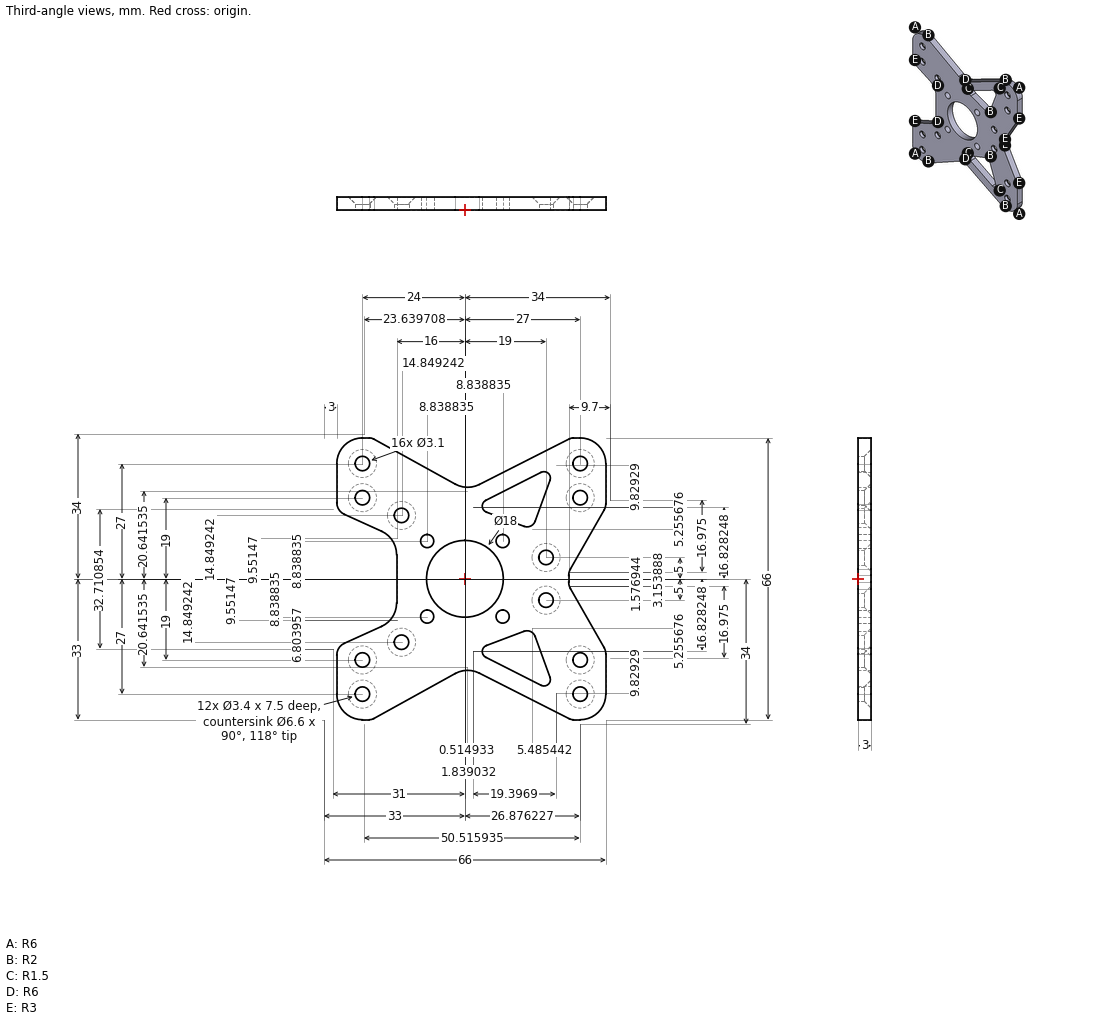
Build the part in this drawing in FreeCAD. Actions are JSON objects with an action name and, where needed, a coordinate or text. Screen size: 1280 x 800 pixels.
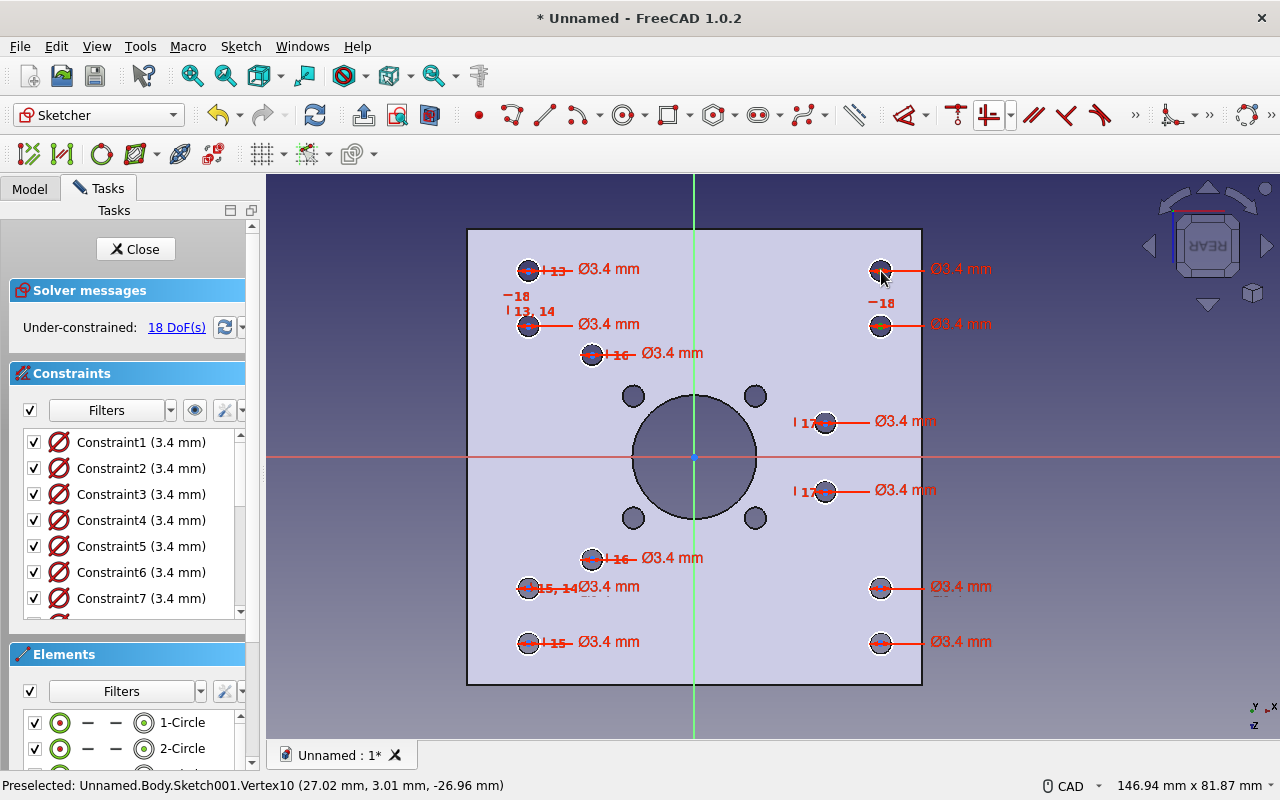
{"action": "key", "text": "v"}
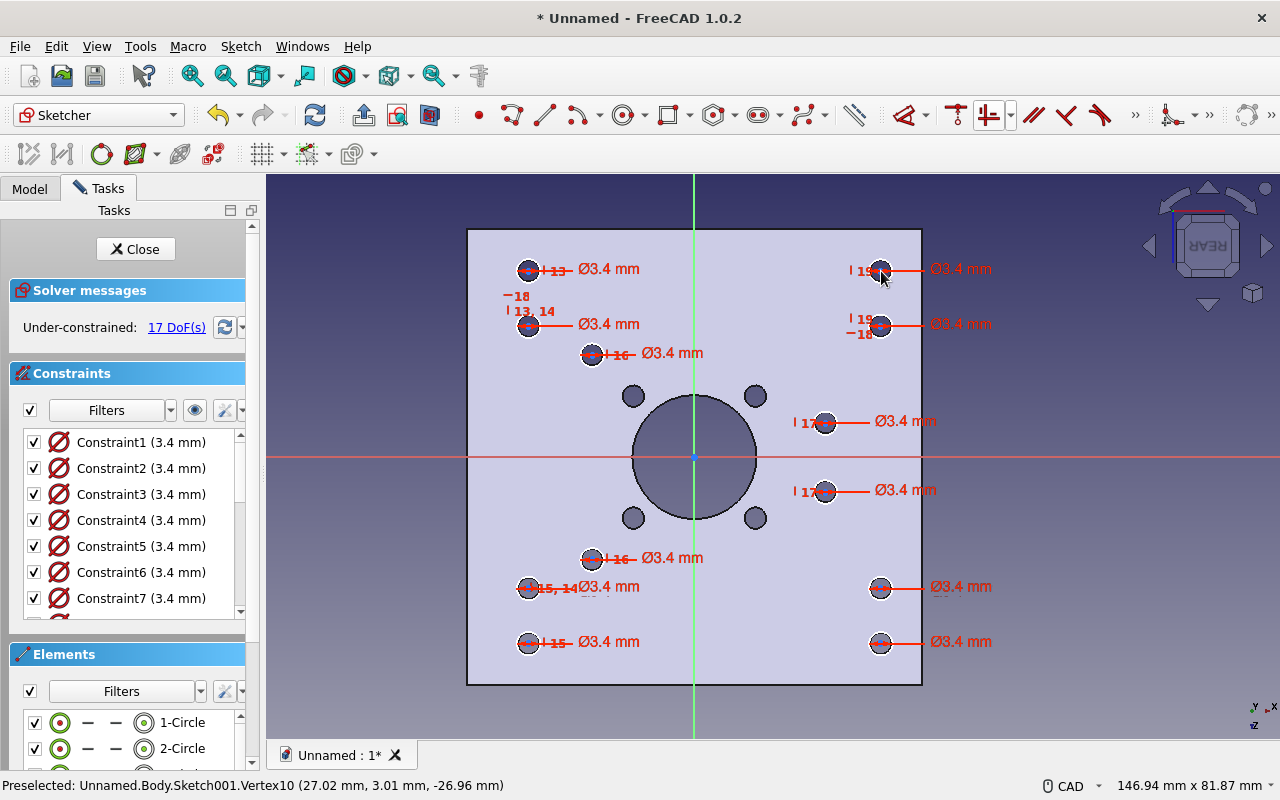
{"action": "left_click", "coordinate": [529, 271]}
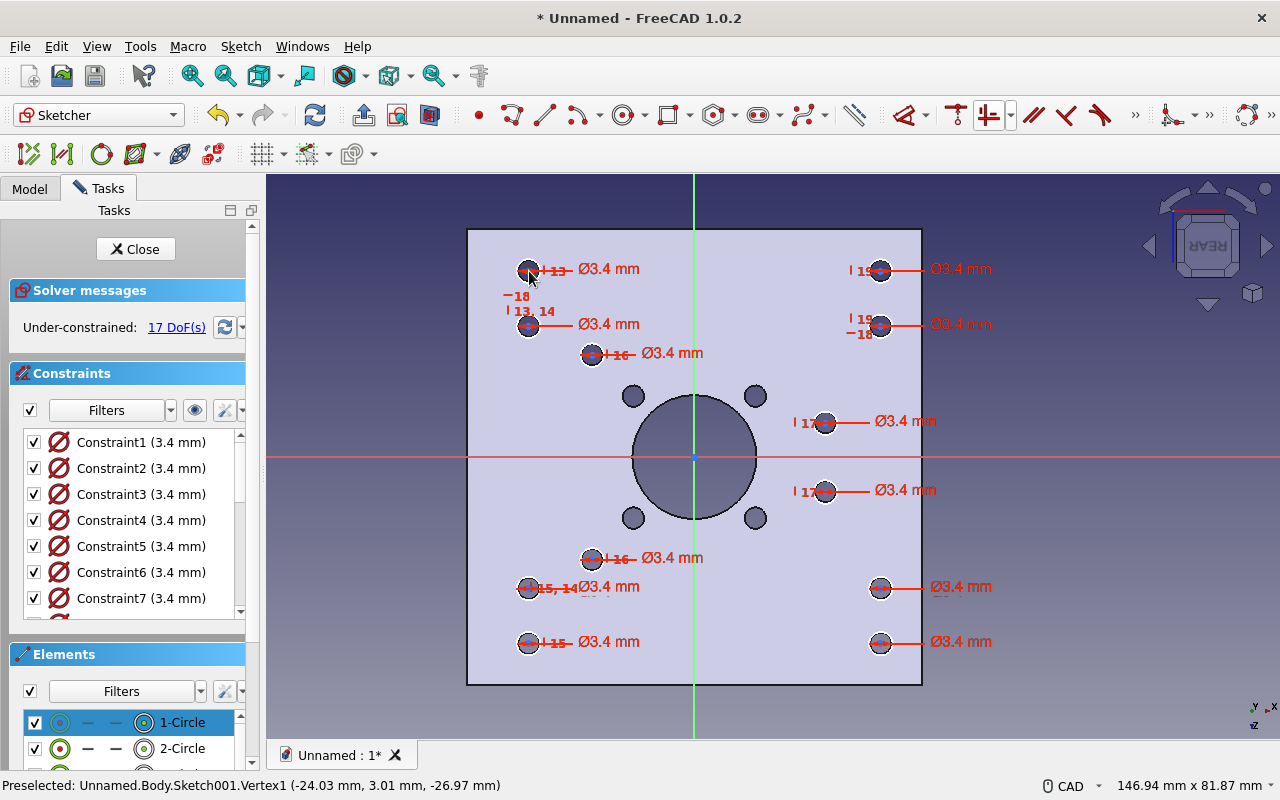
{"action": "left_click", "coordinate": [881, 271]}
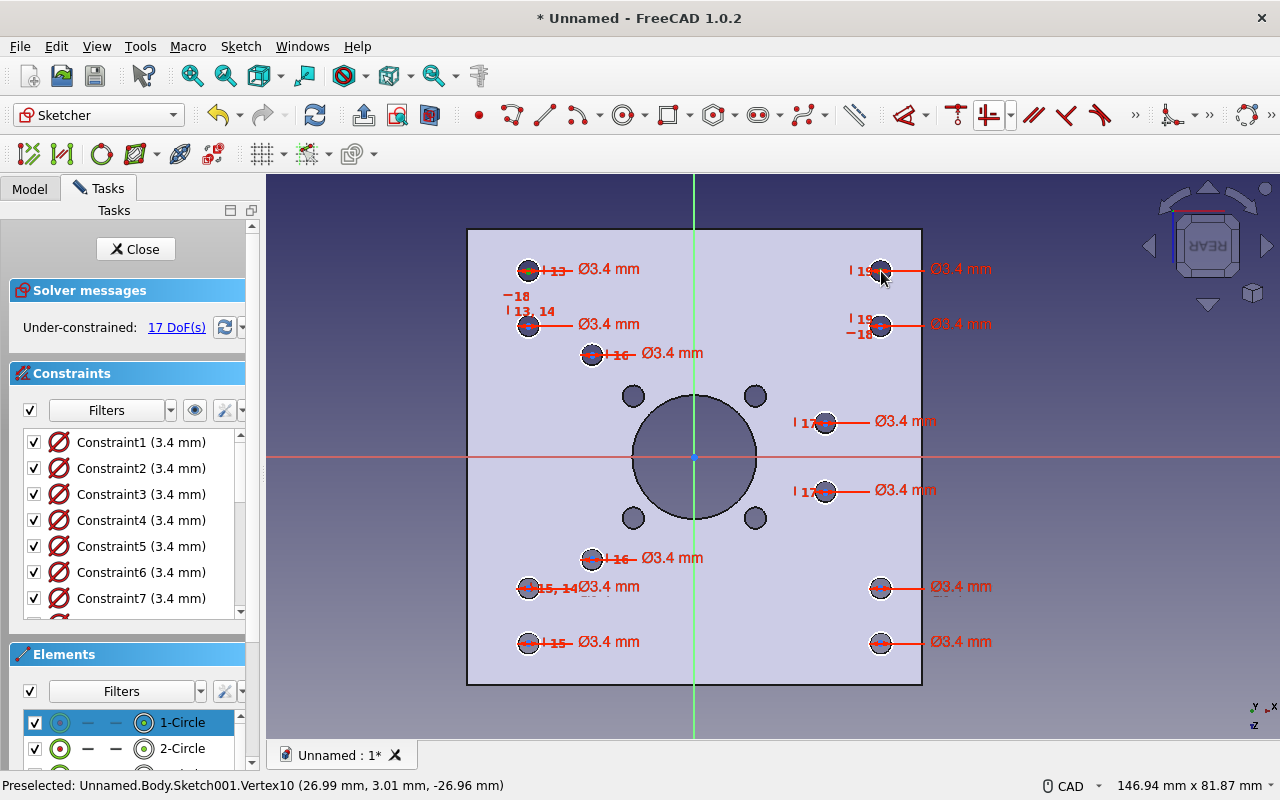
{"action": "left_click", "coordinate": [1010, 116]}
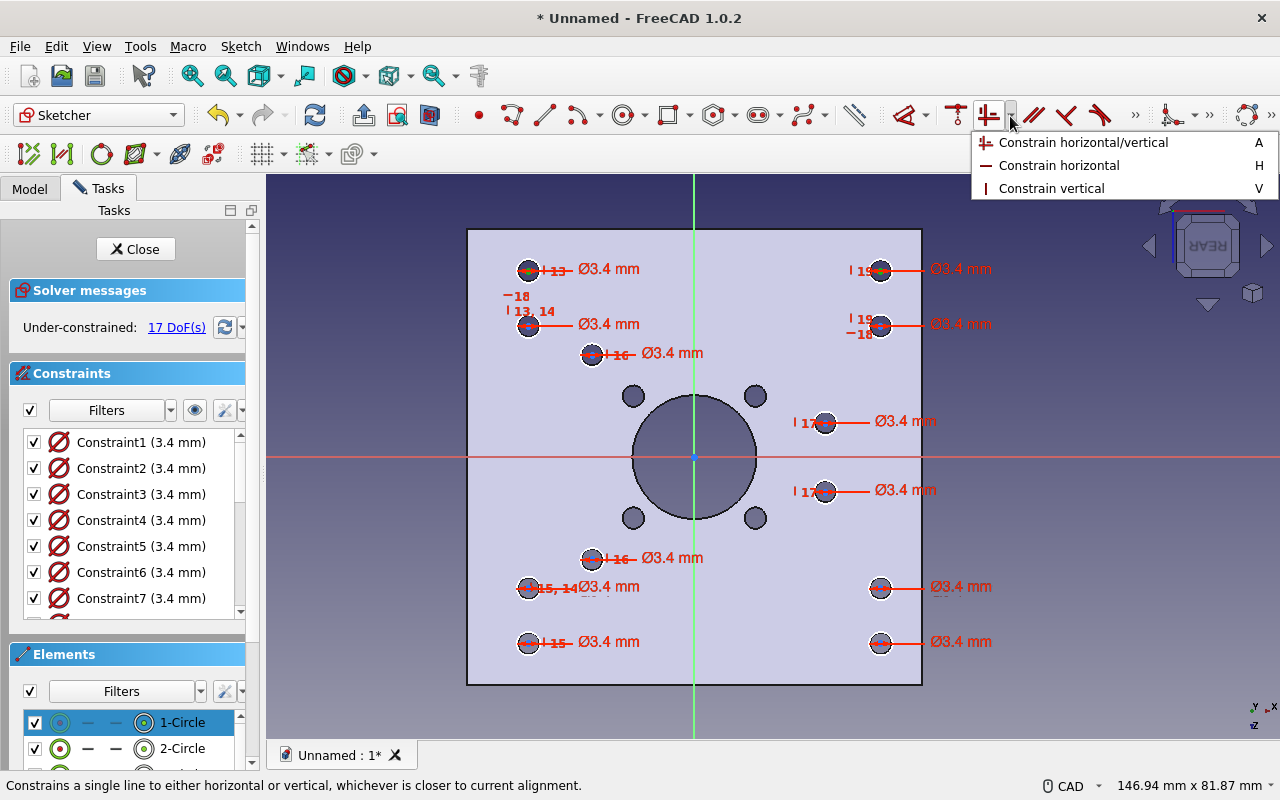
{"action": "left_click", "coordinate": [1125, 166]}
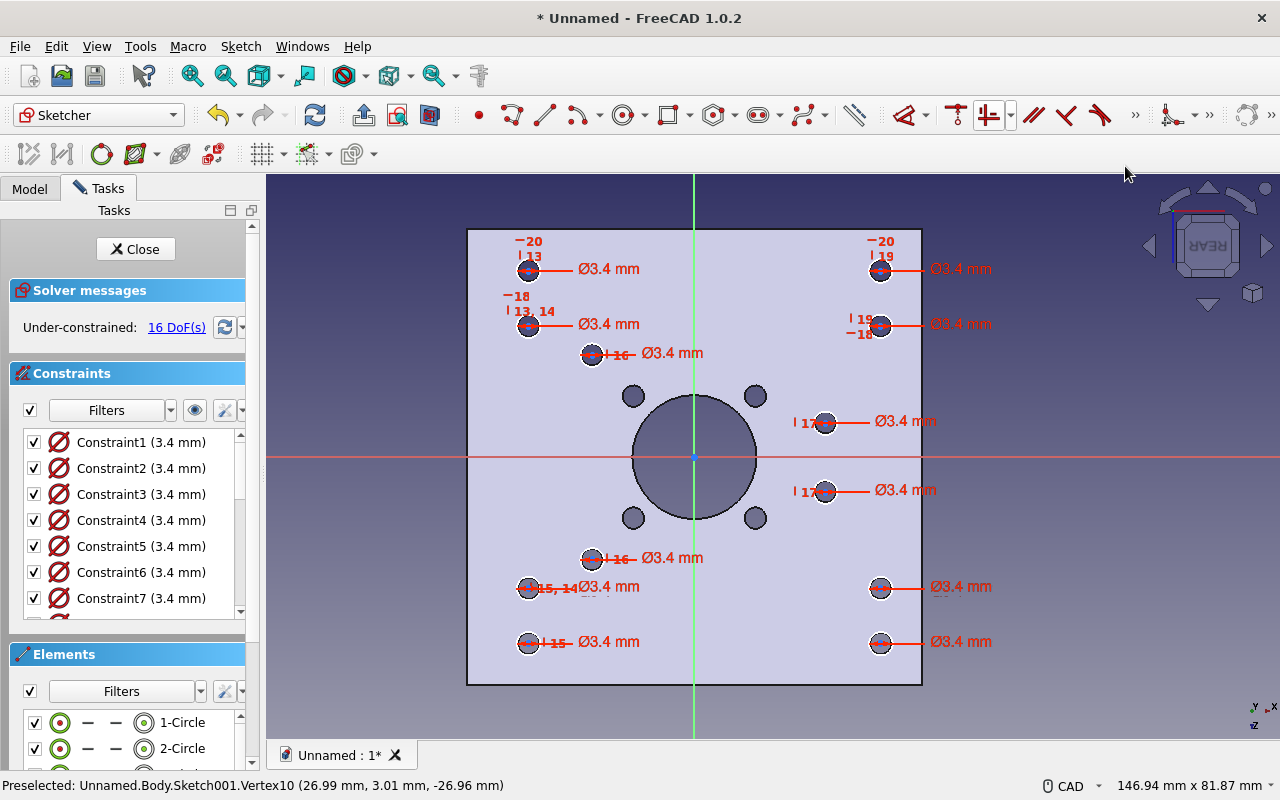
{"action": "left_click", "coordinate": [881, 326]}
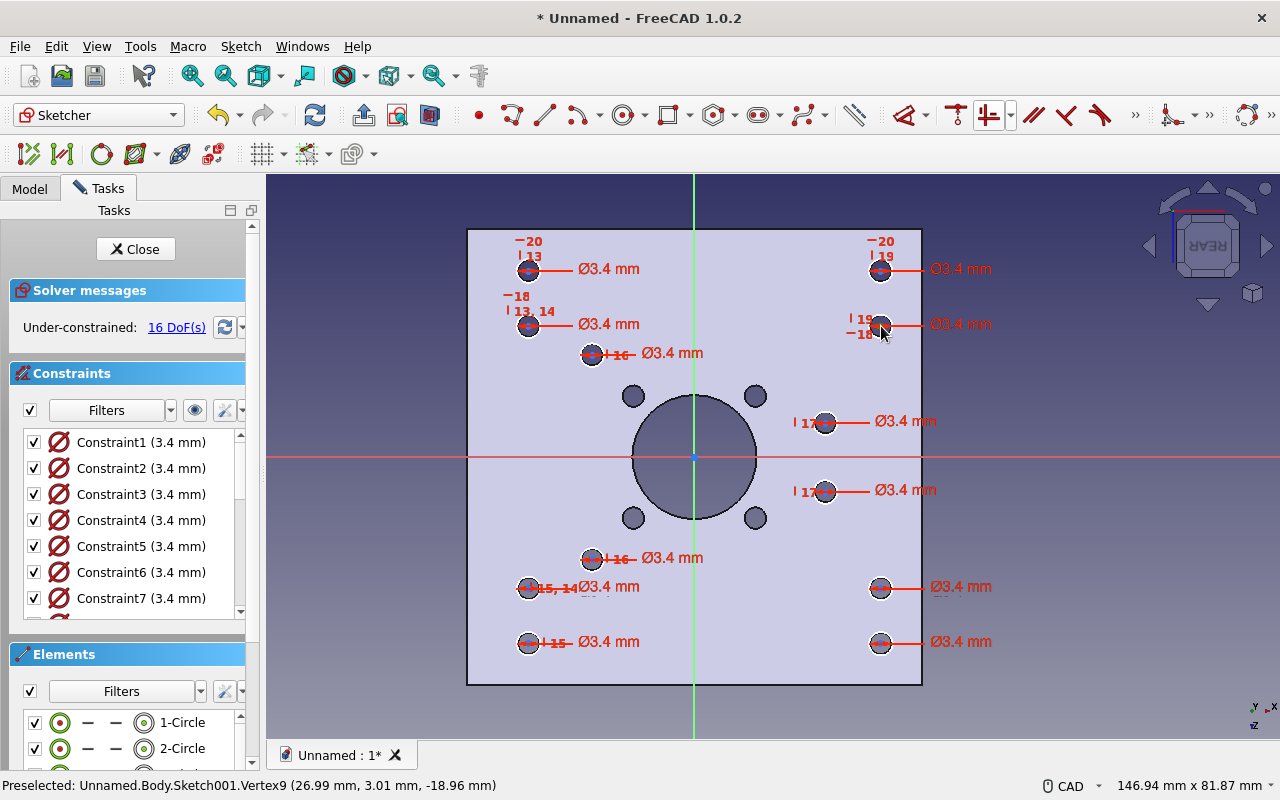
{"action": "left_click", "coordinate": [881, 589]}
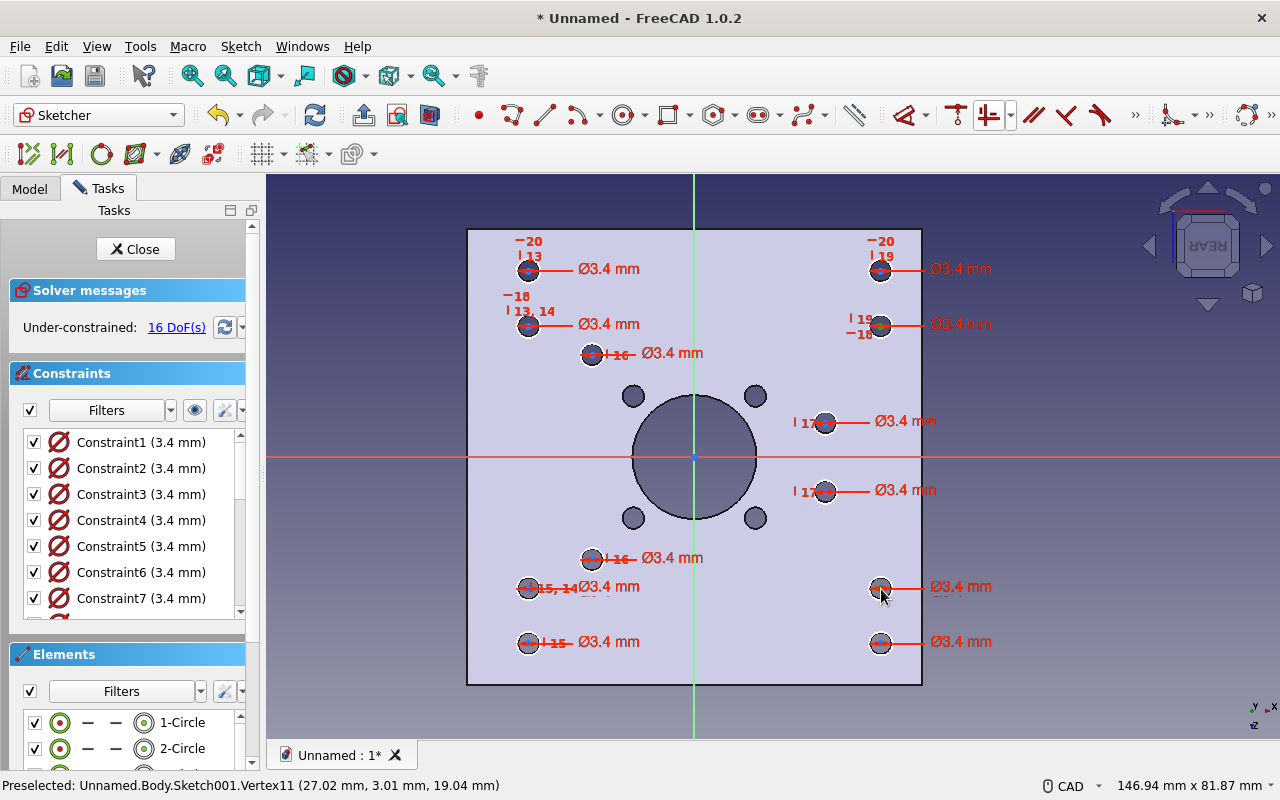
{"action": "key", "text": "v"}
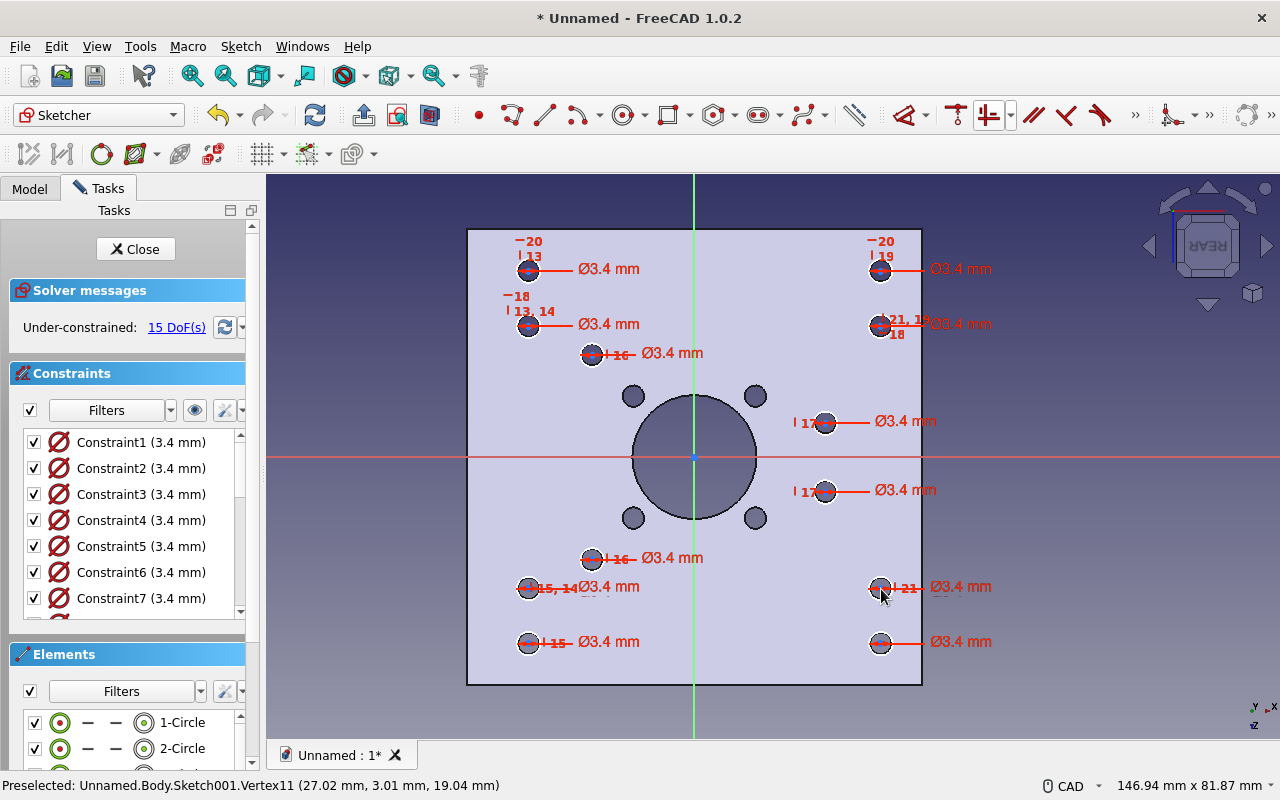
{"action": "left_click", "coordinate": [529, 589]}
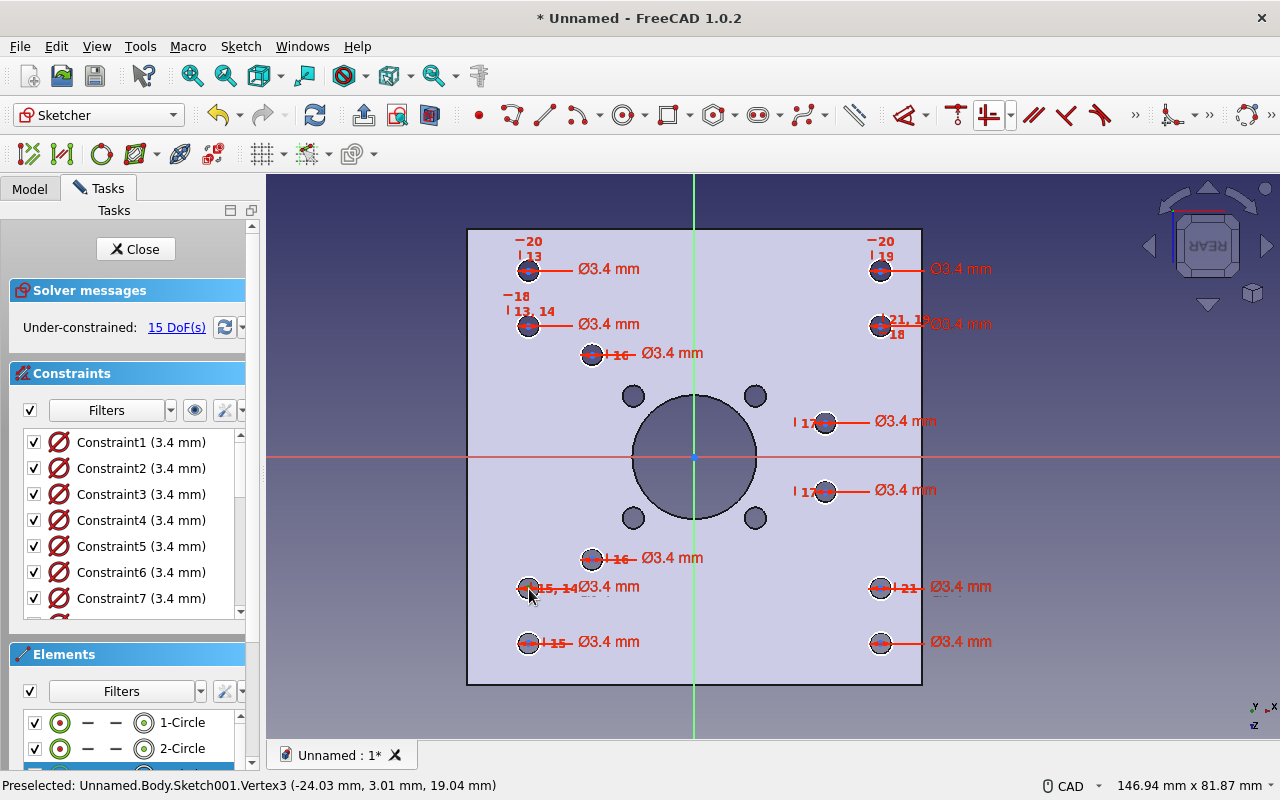
{"action": "left_click", "coordinate": [881, 589]}